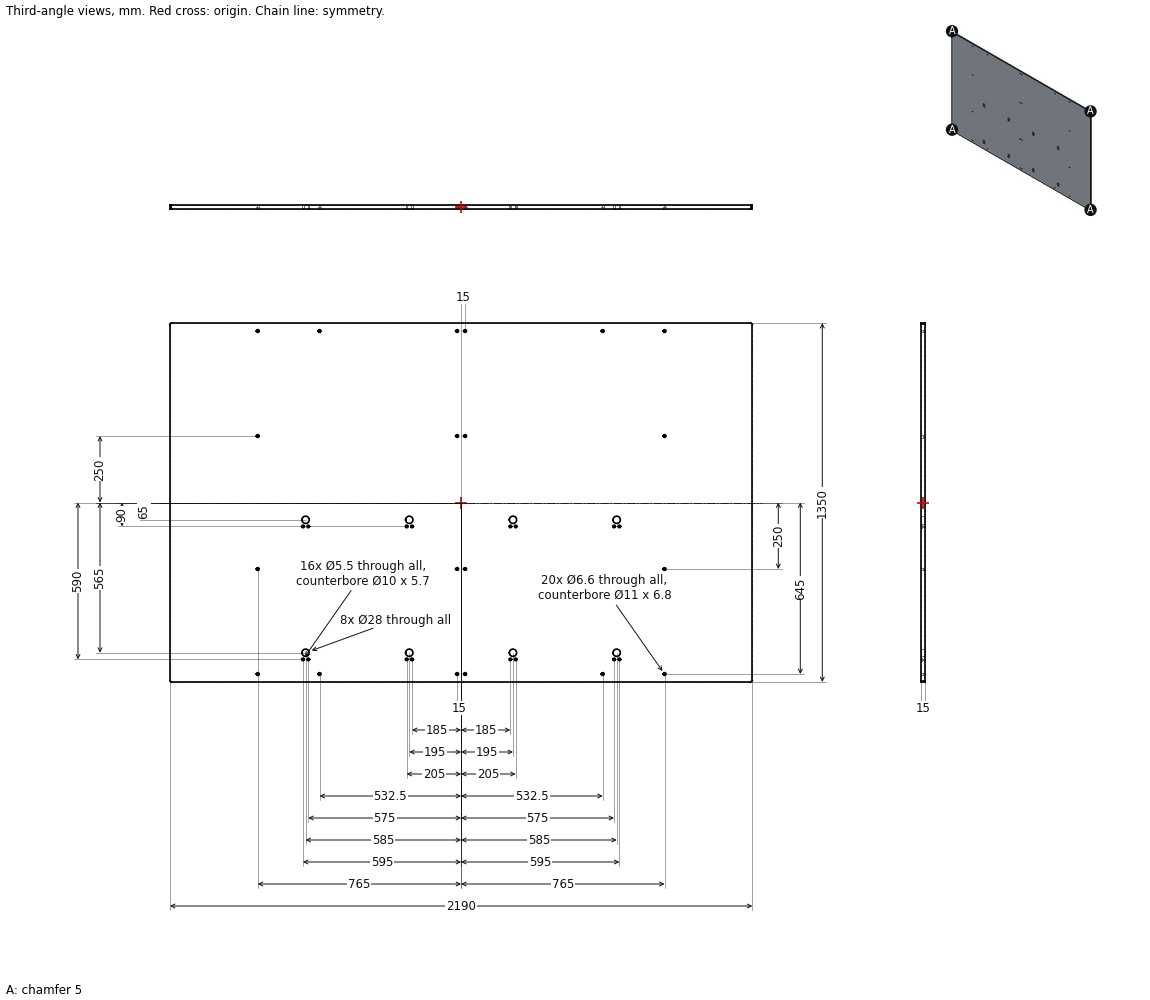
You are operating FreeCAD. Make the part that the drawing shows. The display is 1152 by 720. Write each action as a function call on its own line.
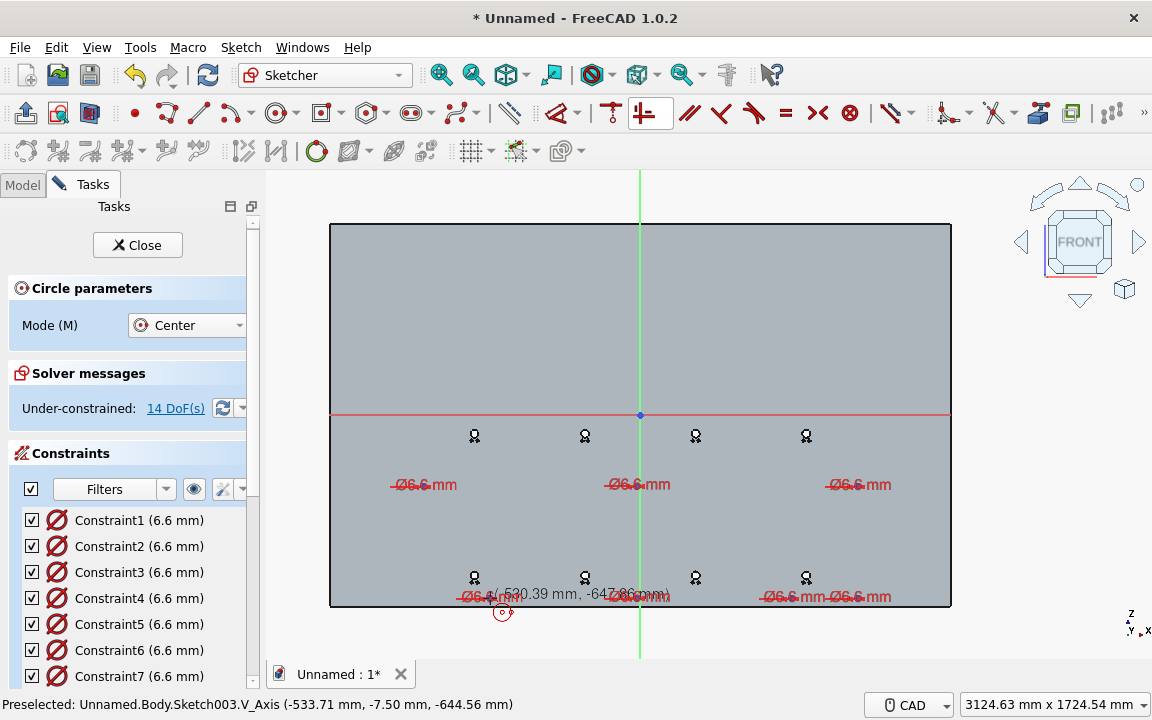
scroll(423, 598, up, 16)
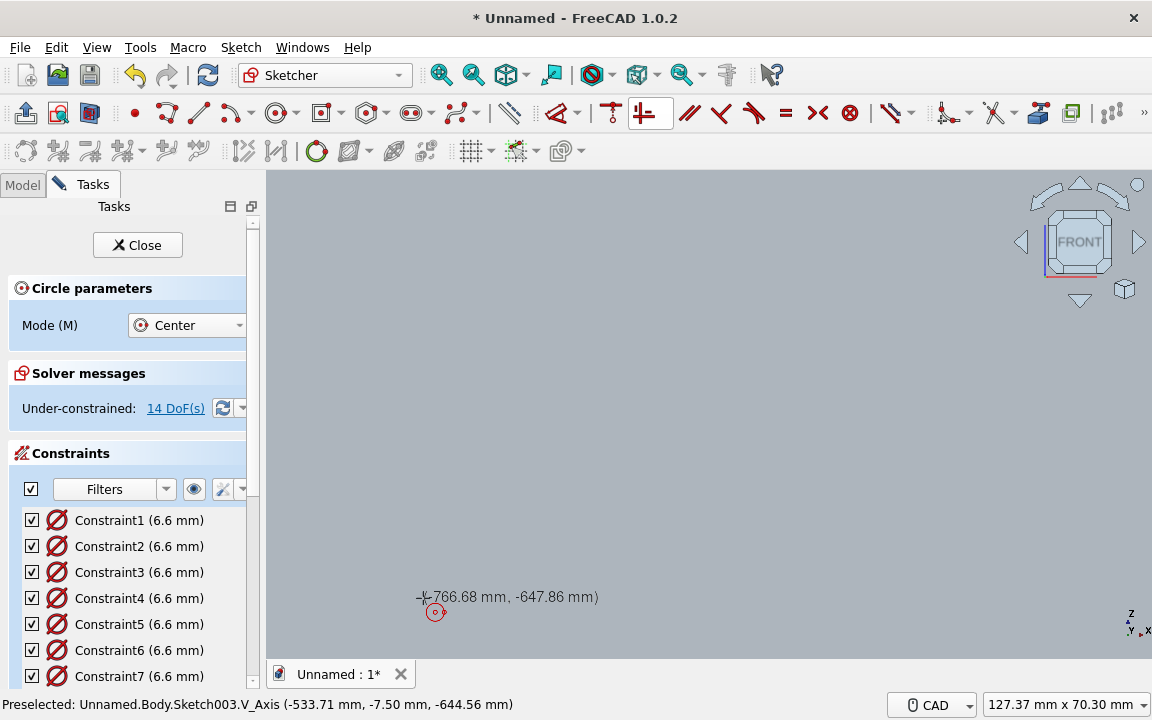
scroll(423, 598, down, 16)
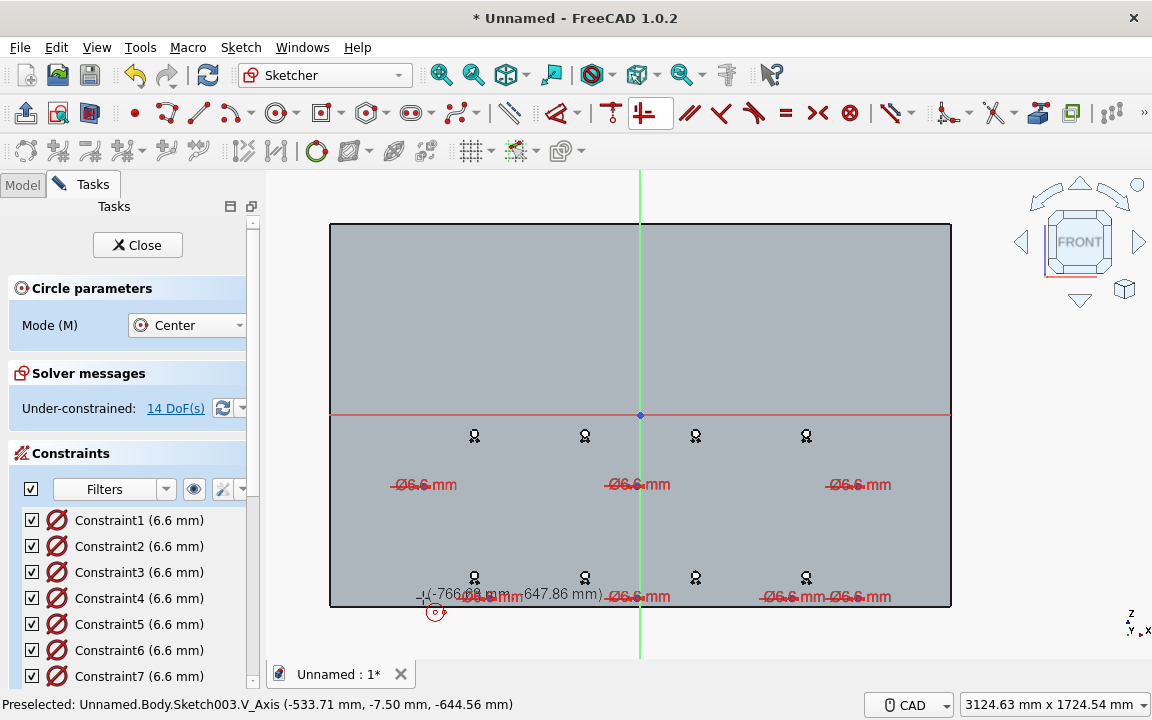
click(423, 598)
move(424, 598)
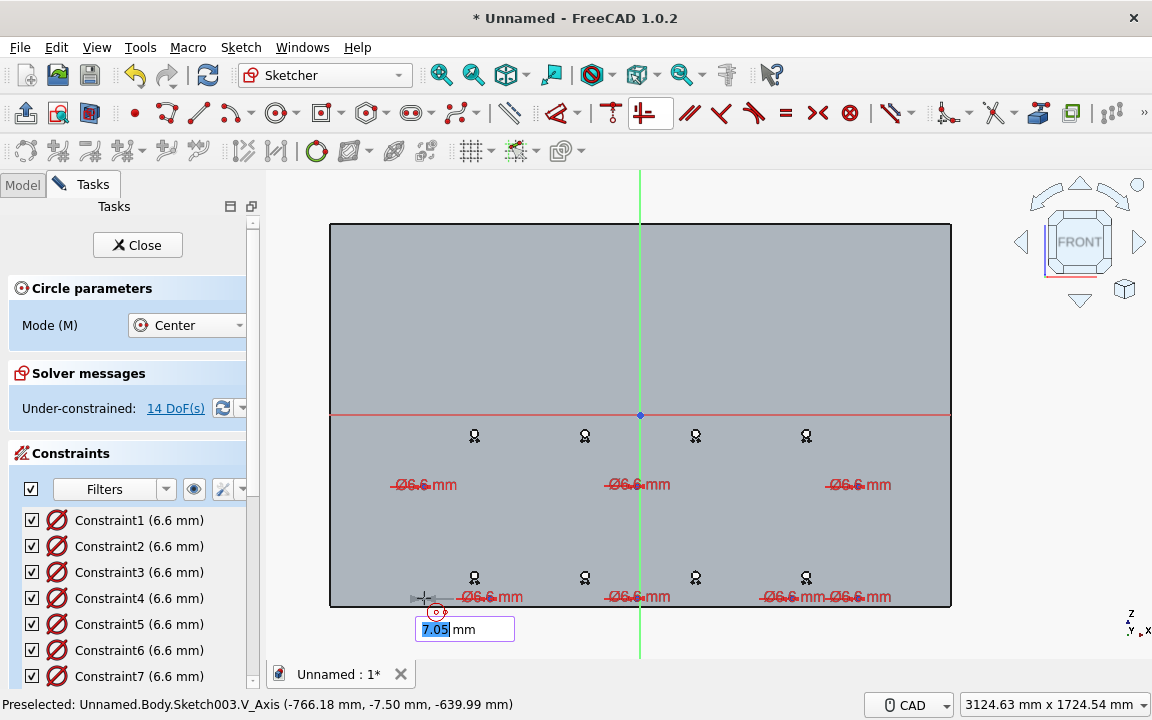
text(6.6)
key(Return)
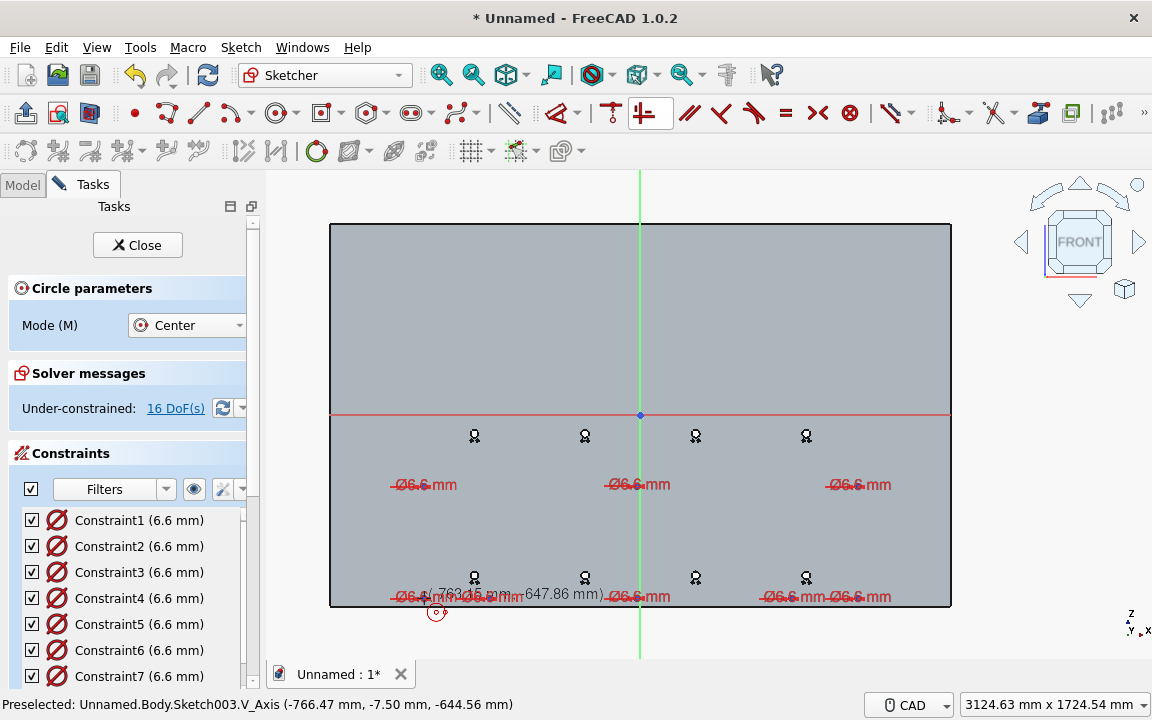
scroll(423, 232, up, 16)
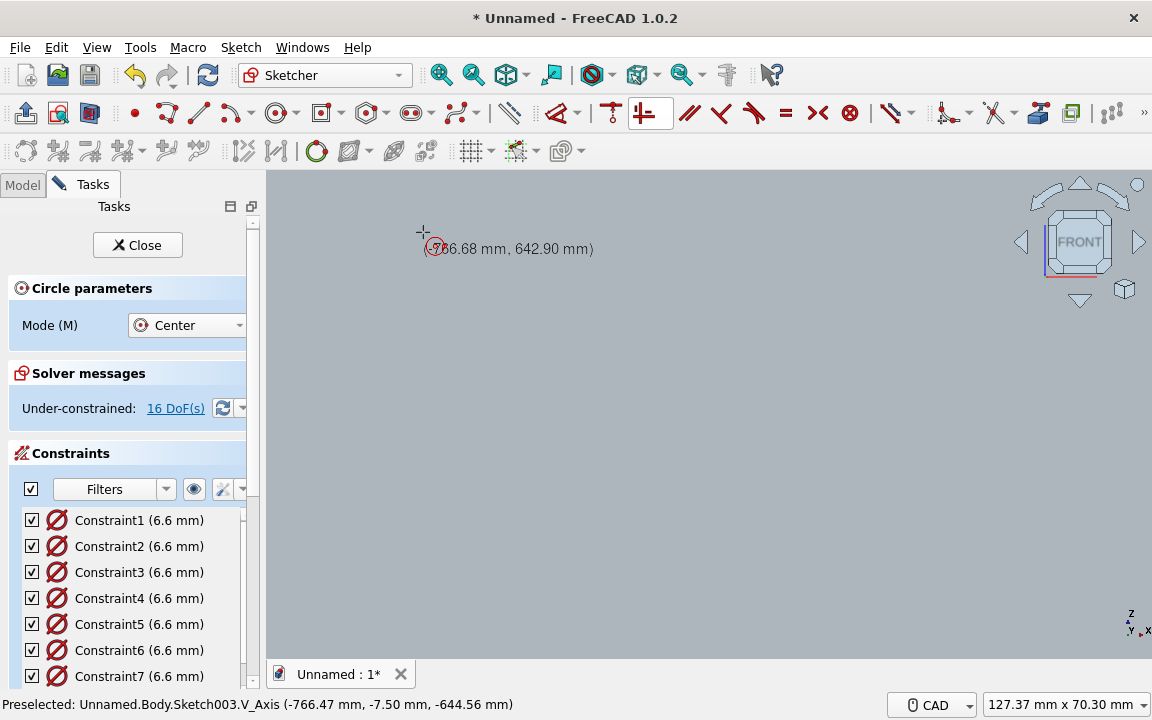
scroll(423, 231, down, 16)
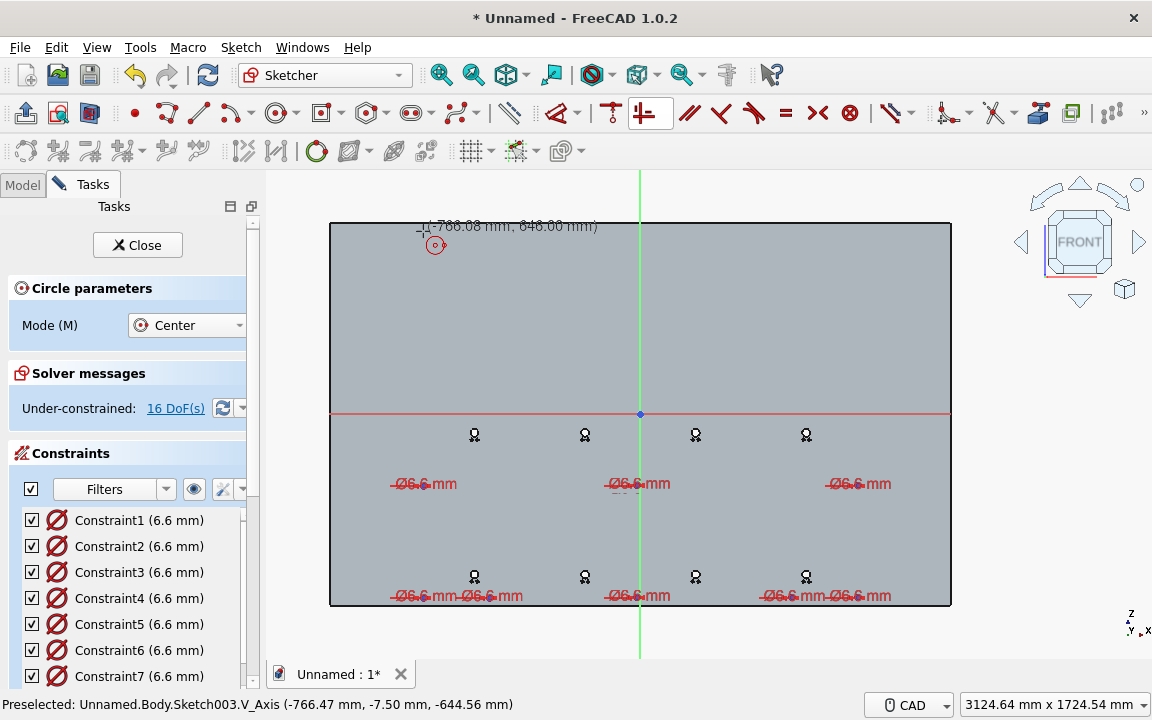
click(423, 231)
move(424, 231)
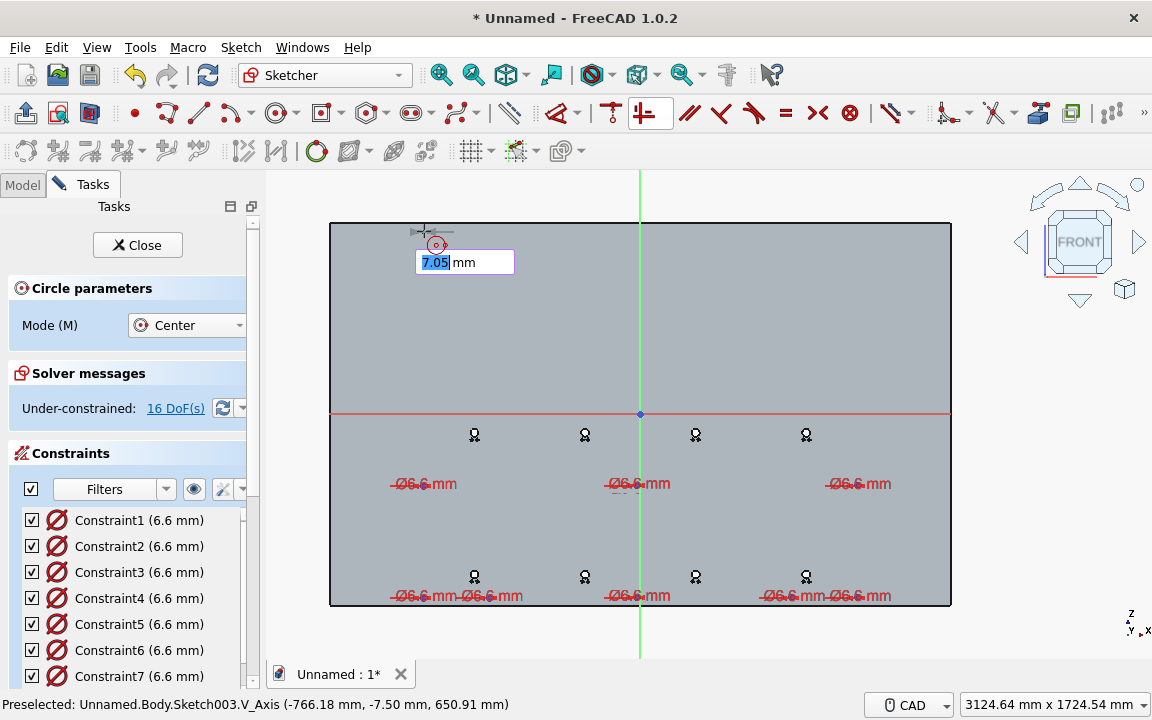
text(6.6)
key(Return)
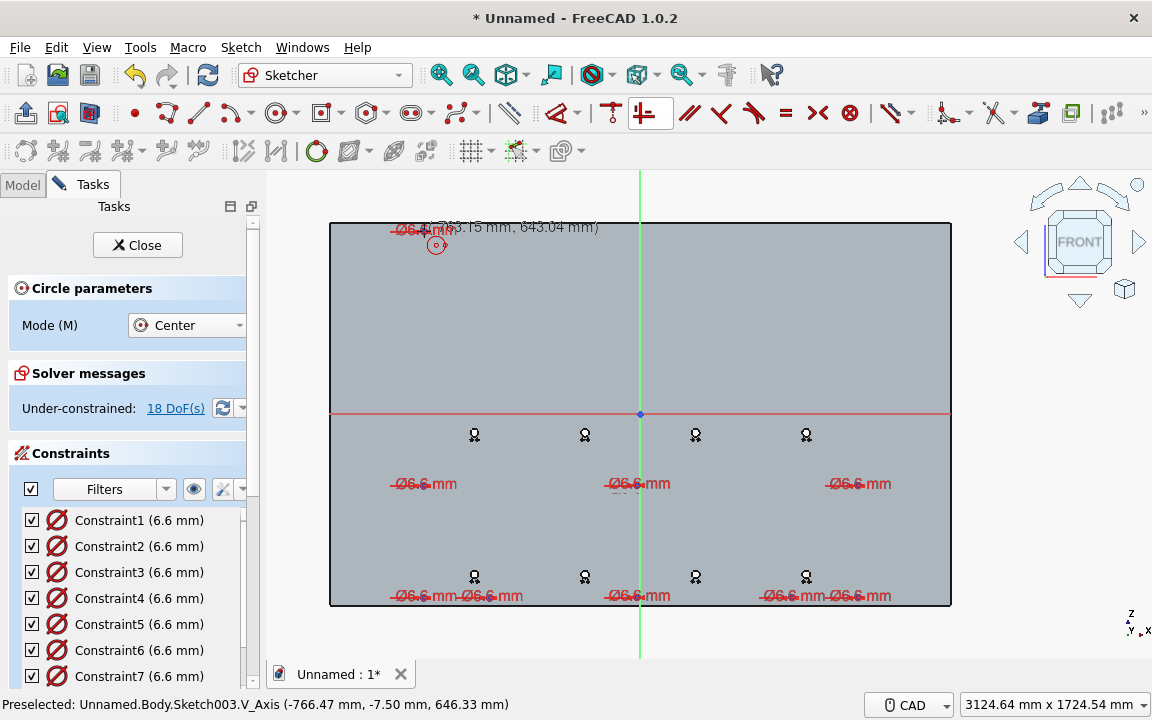
scroll(489, 231, up, 16)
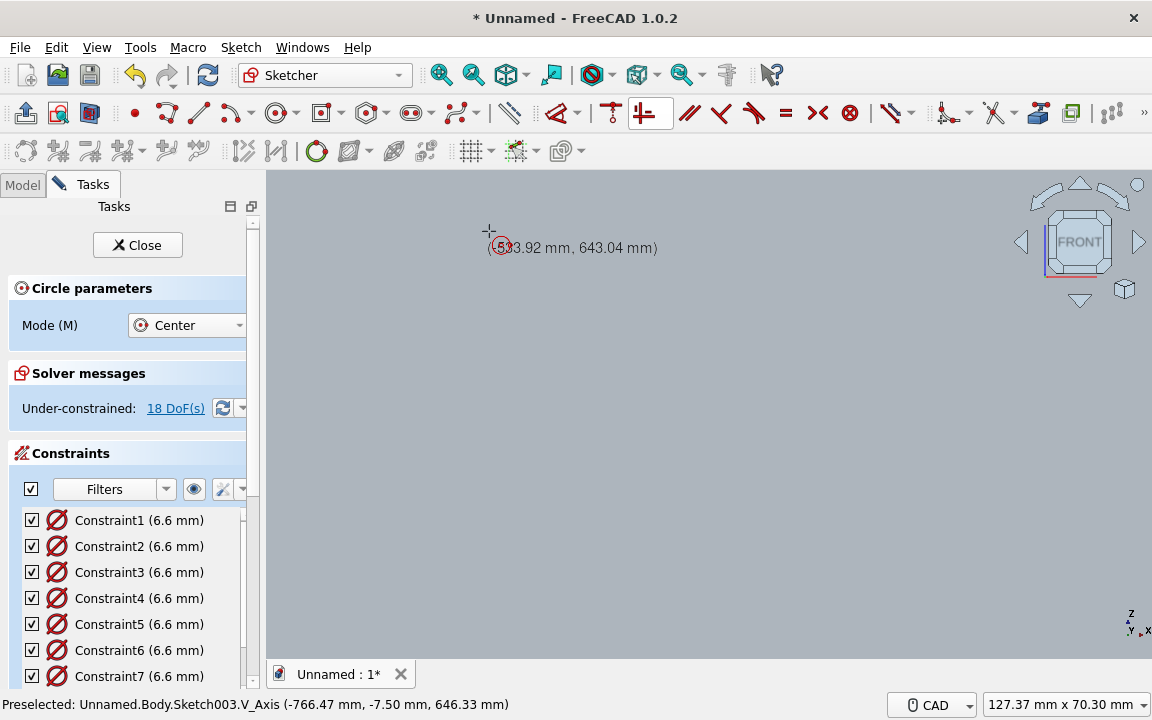
scroll(489, 231, down, 16)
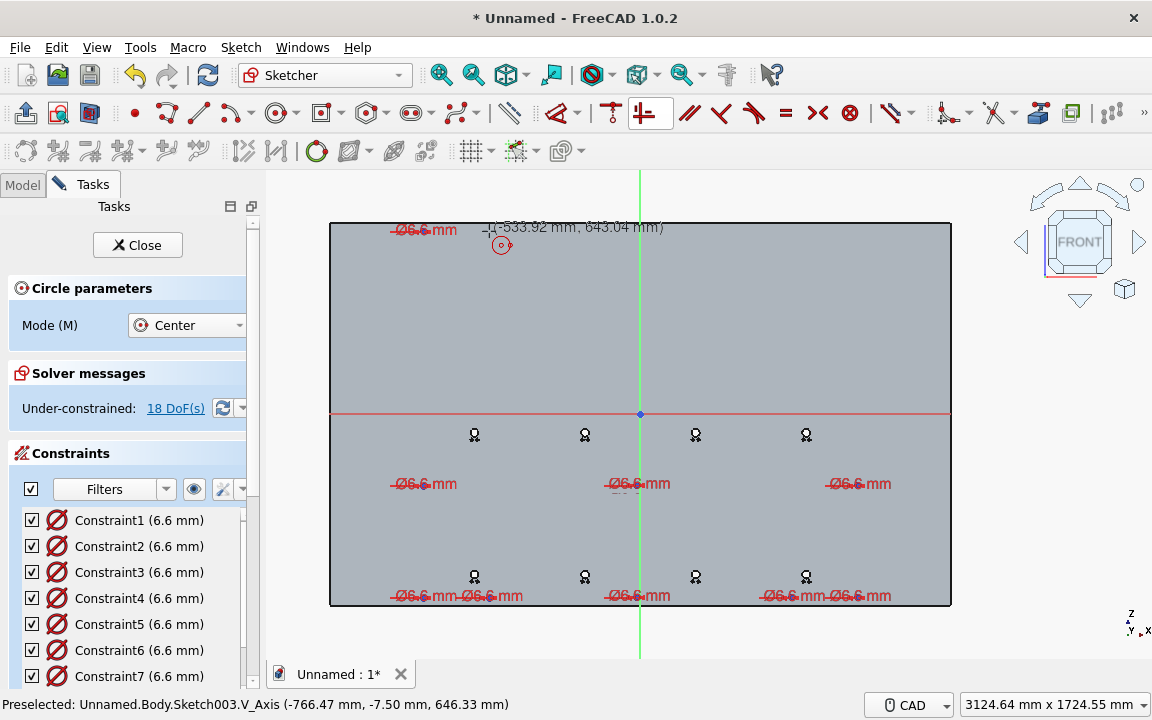
click(489, 231)
move(490, 231)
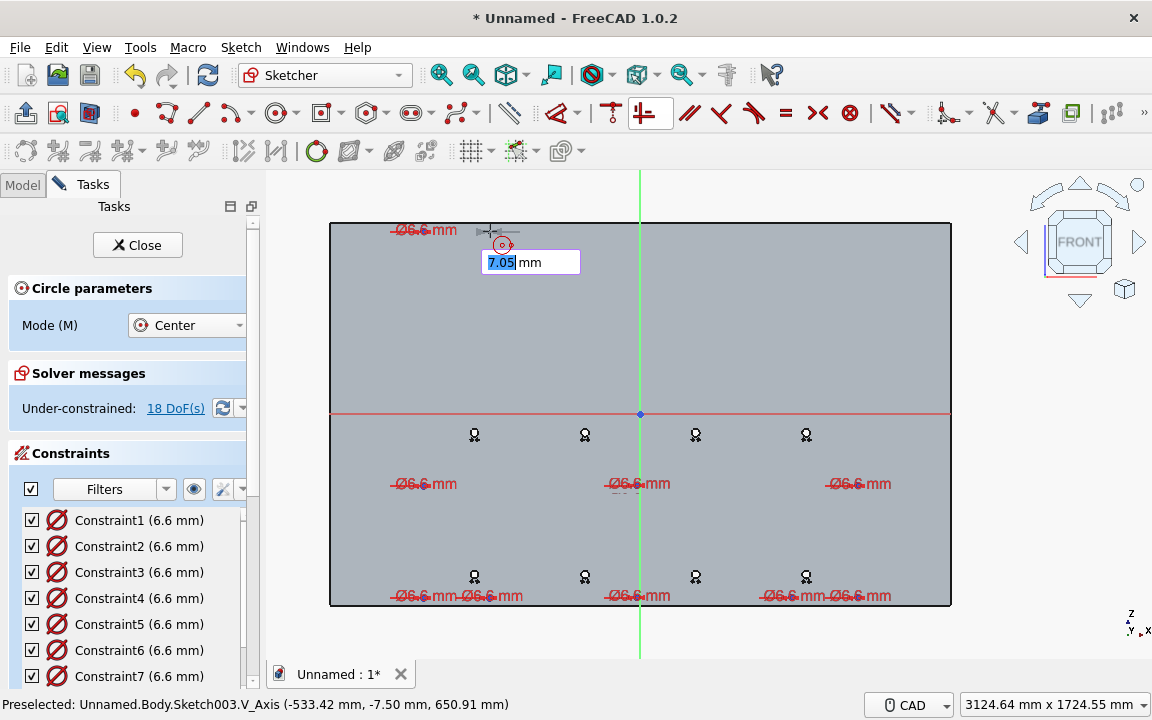
text(6.6)
key(Return)